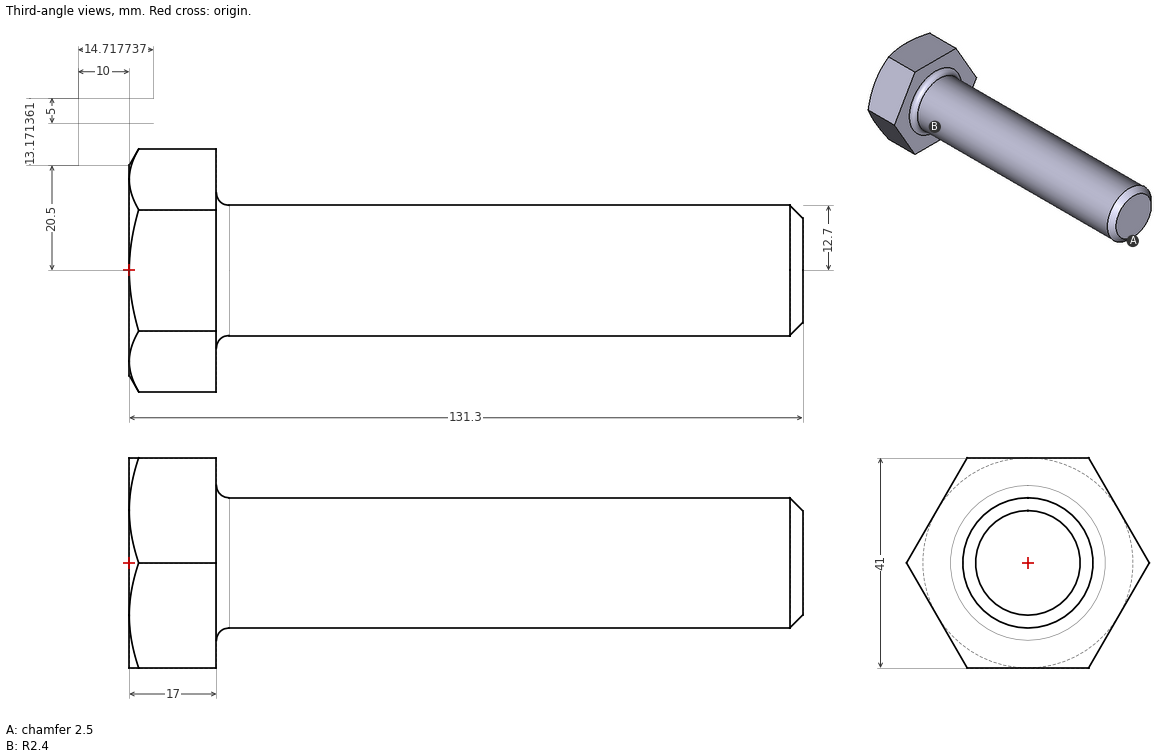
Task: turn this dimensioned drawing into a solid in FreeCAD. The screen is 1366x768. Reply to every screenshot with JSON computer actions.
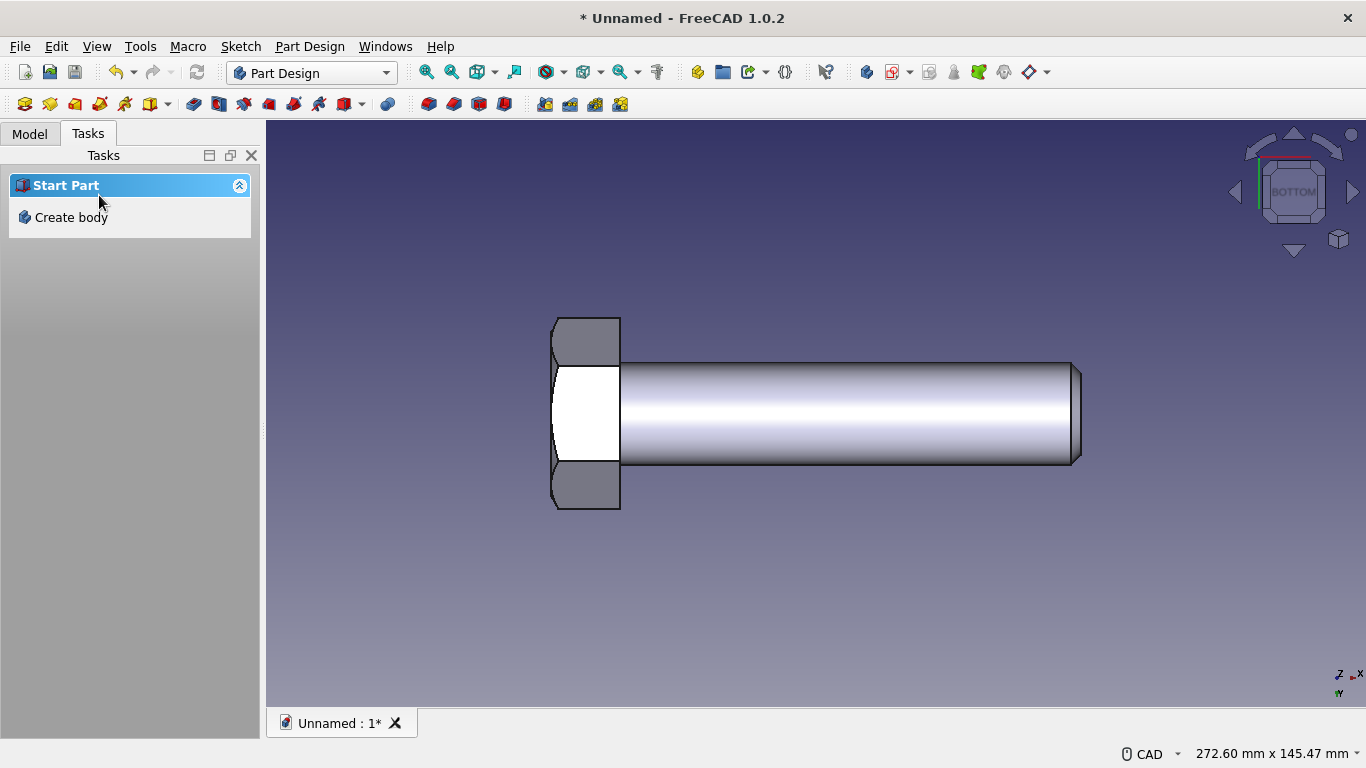
{"action": "key", "text": "4"}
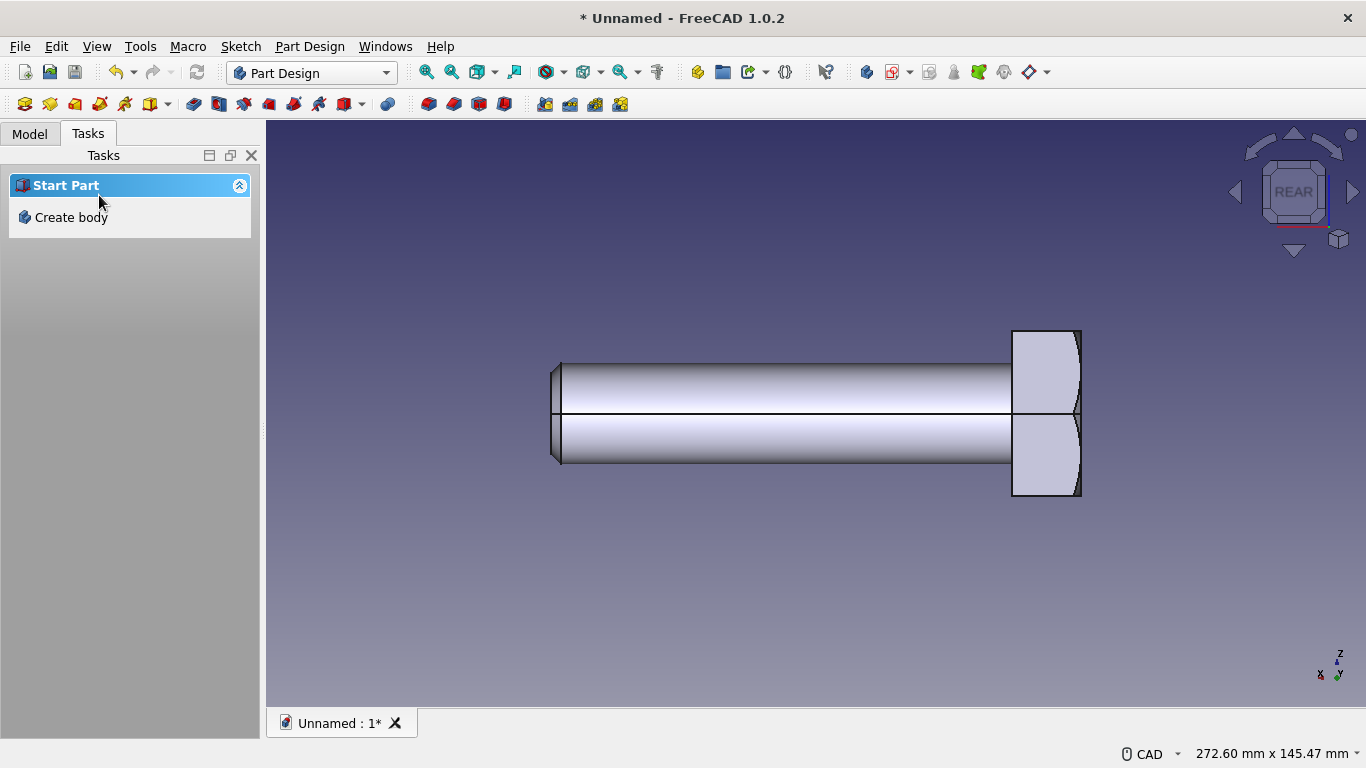
{"action": "key", "text": "6"}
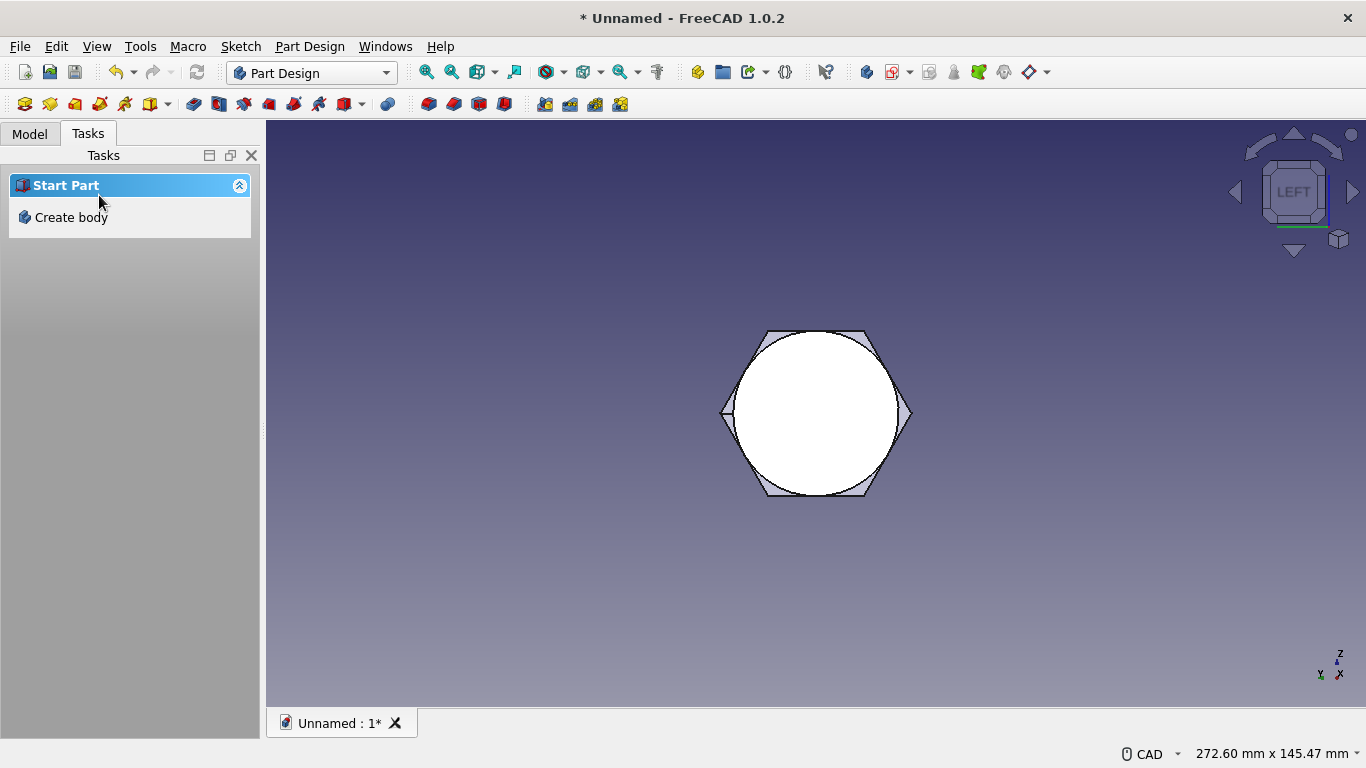
{"action": "key", "text": "v f"}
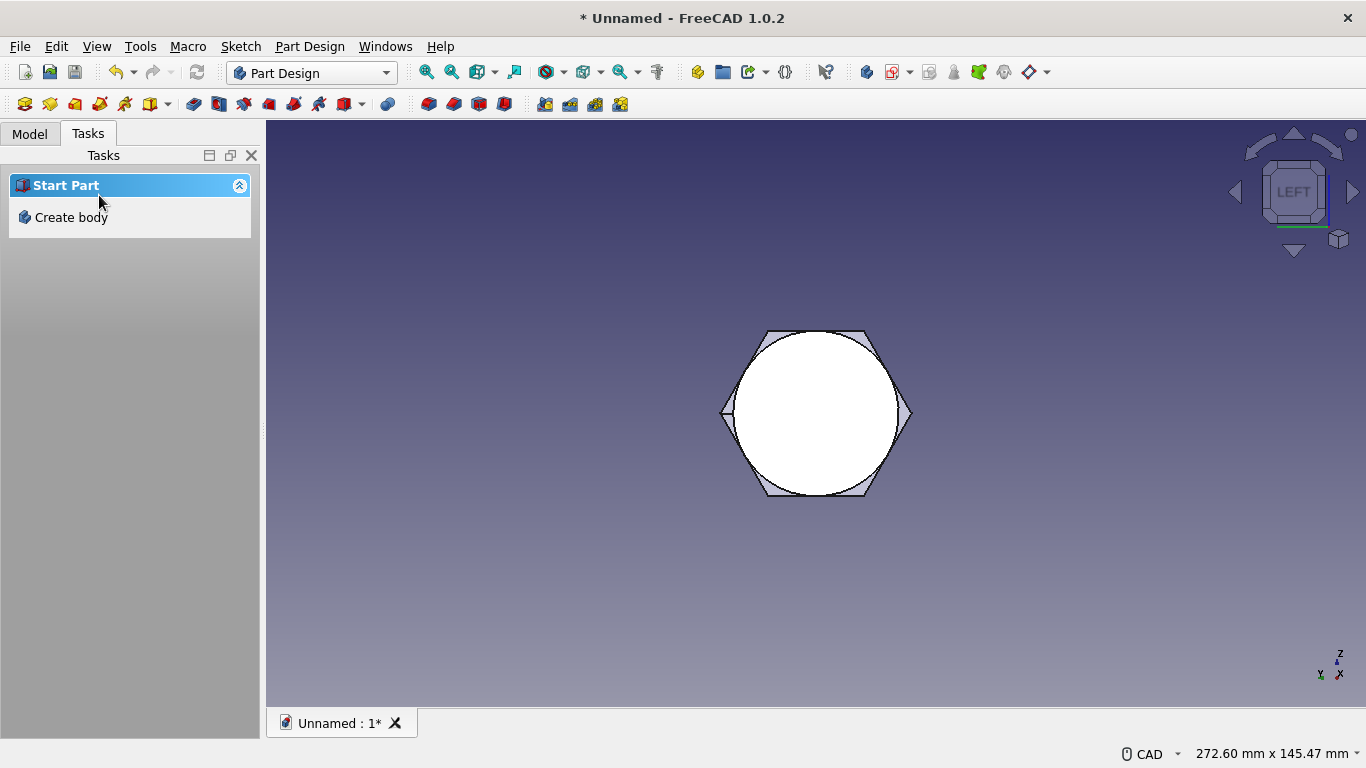
{"action": "key", "text": "v 3"}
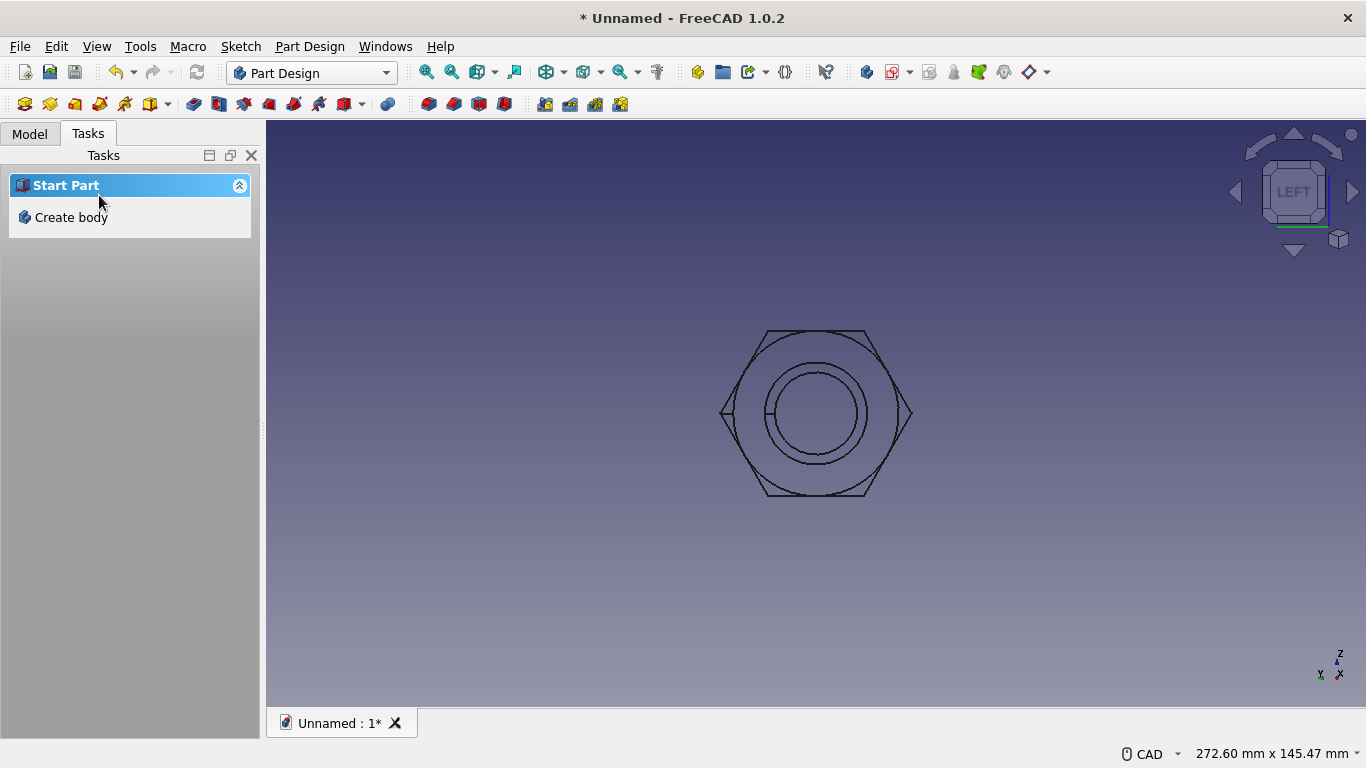
{"action": "key", "text": "0"}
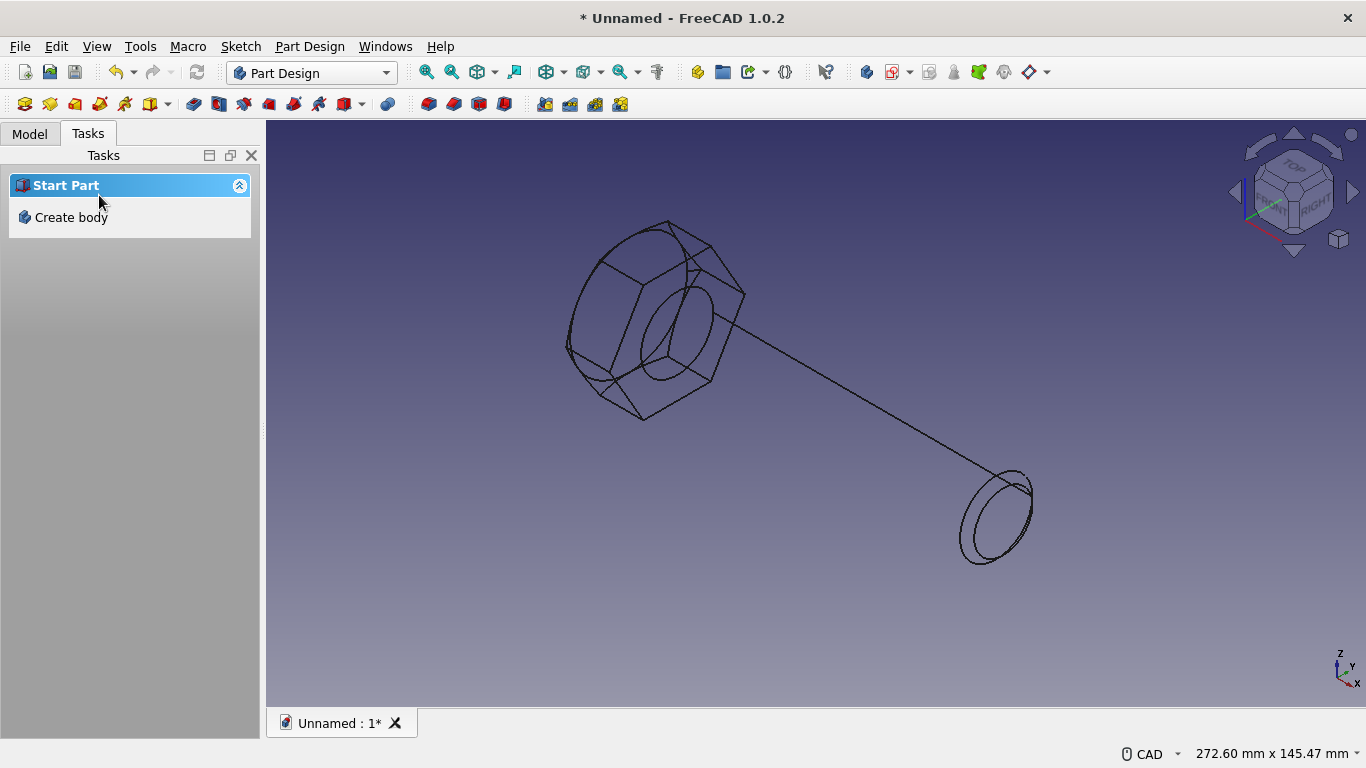
{"action": "left_click", "coordinate": [641, 353]}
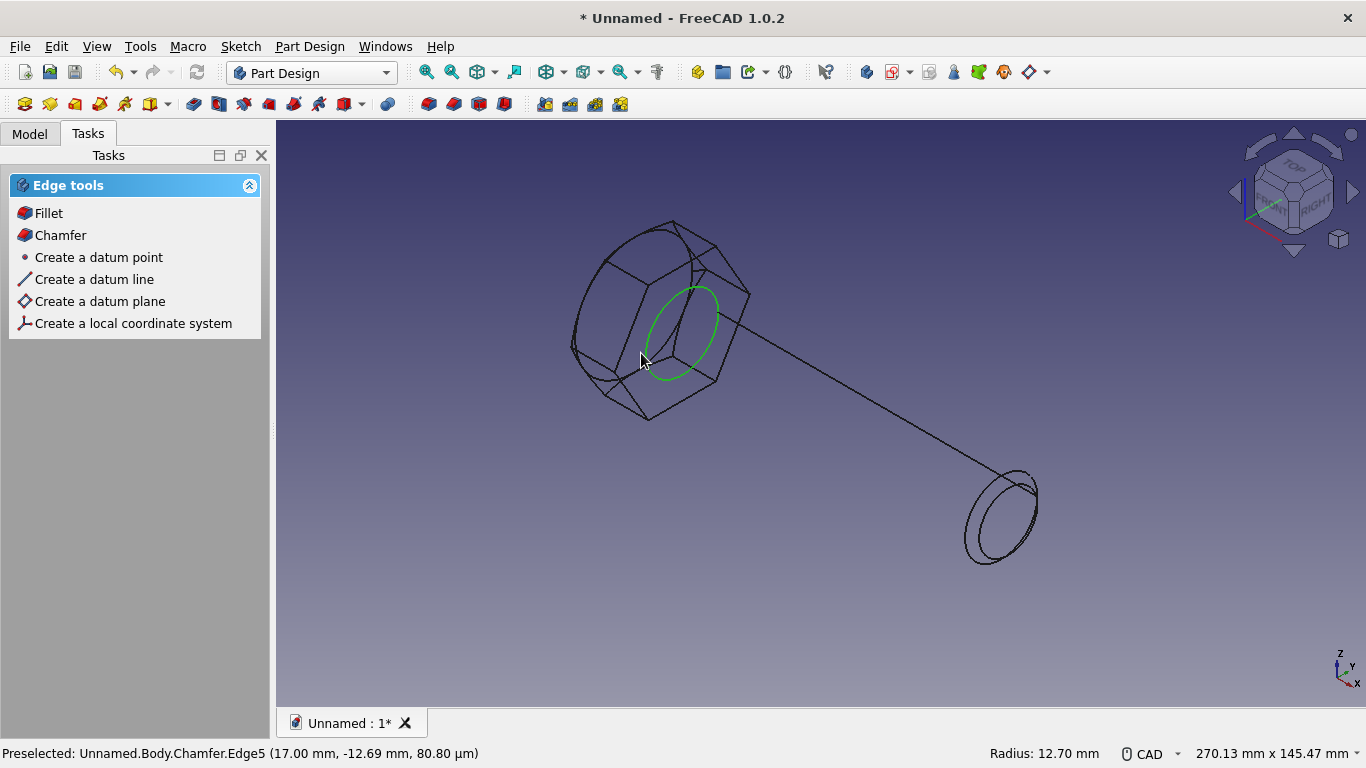
{"action": "key", "text": "v 1"}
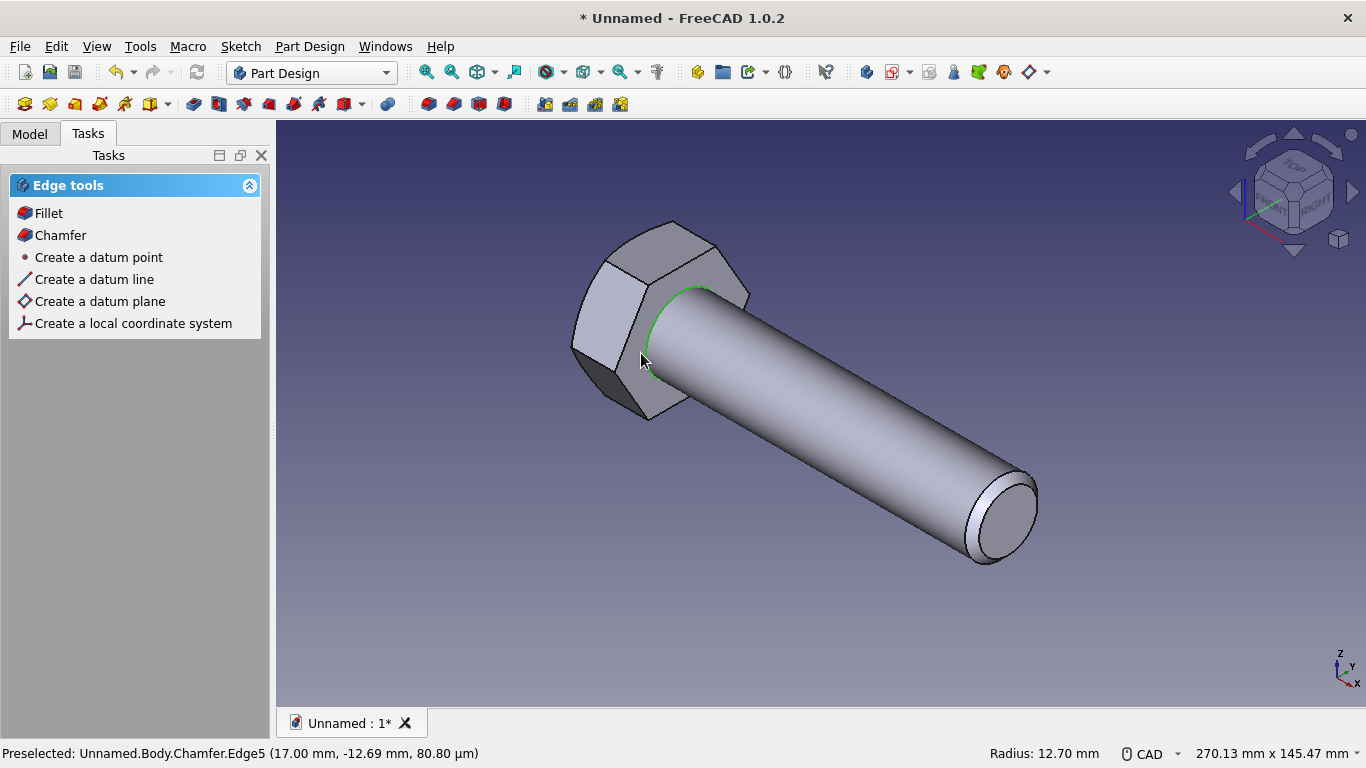
{"action": "left_click", "coordinate": [429, 104]}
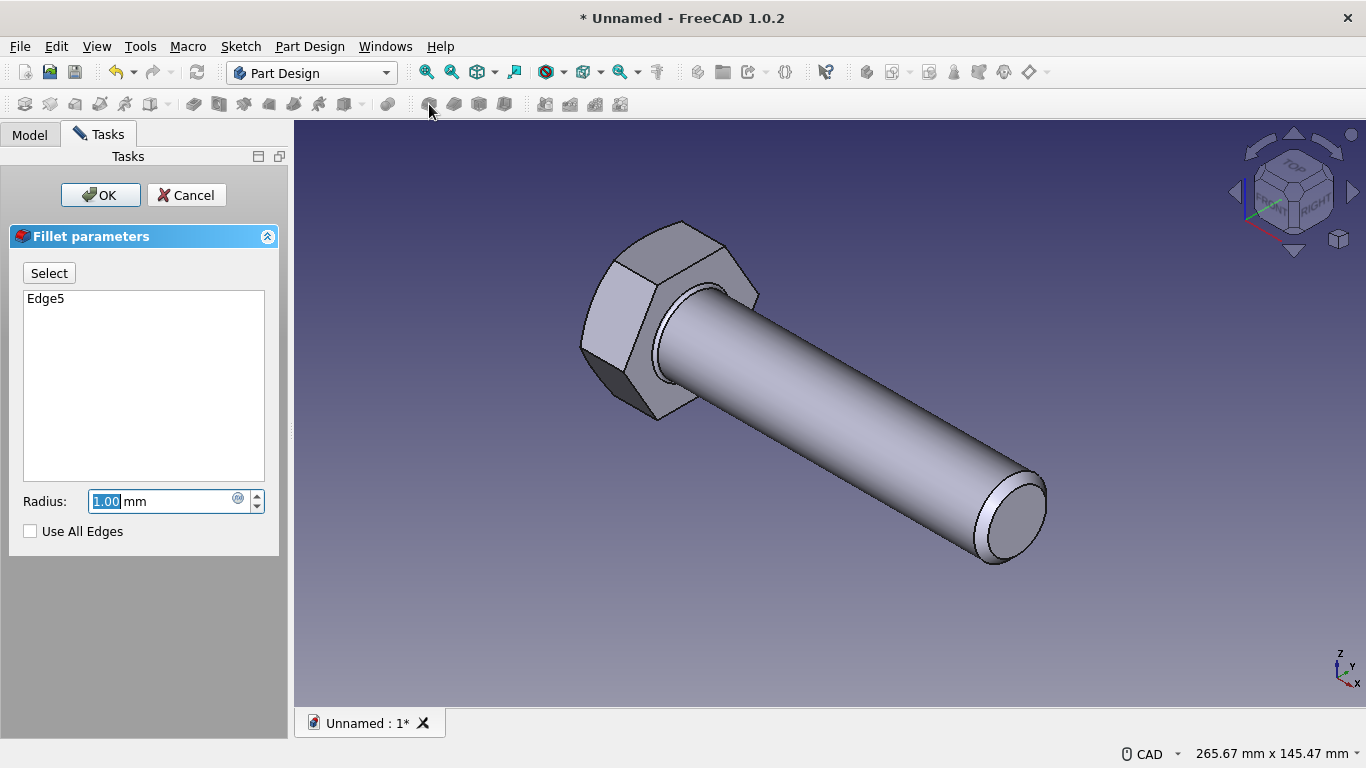
{"action": "type", "text": "2.4"}
{"action": "key", "text": "Tab"}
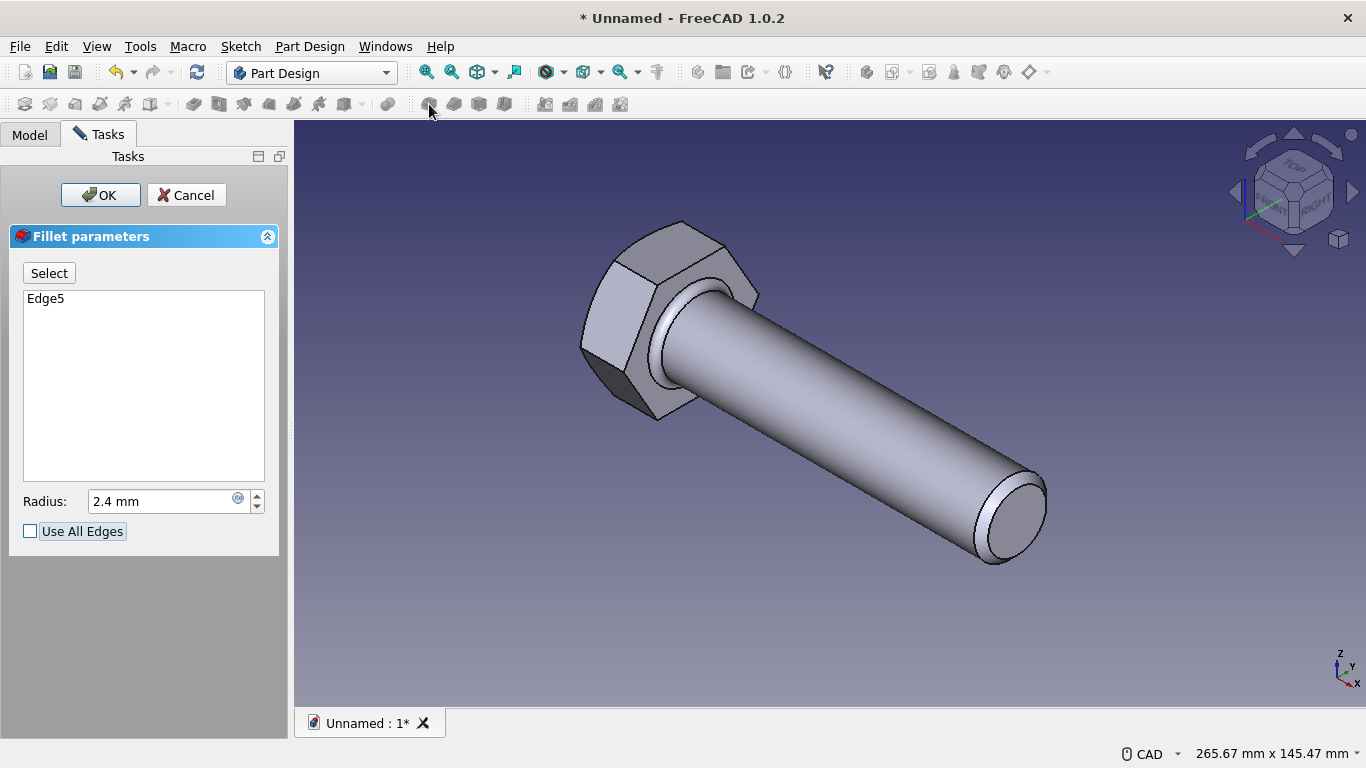
{"action": "left_click", "coordinate": [101, 195]}